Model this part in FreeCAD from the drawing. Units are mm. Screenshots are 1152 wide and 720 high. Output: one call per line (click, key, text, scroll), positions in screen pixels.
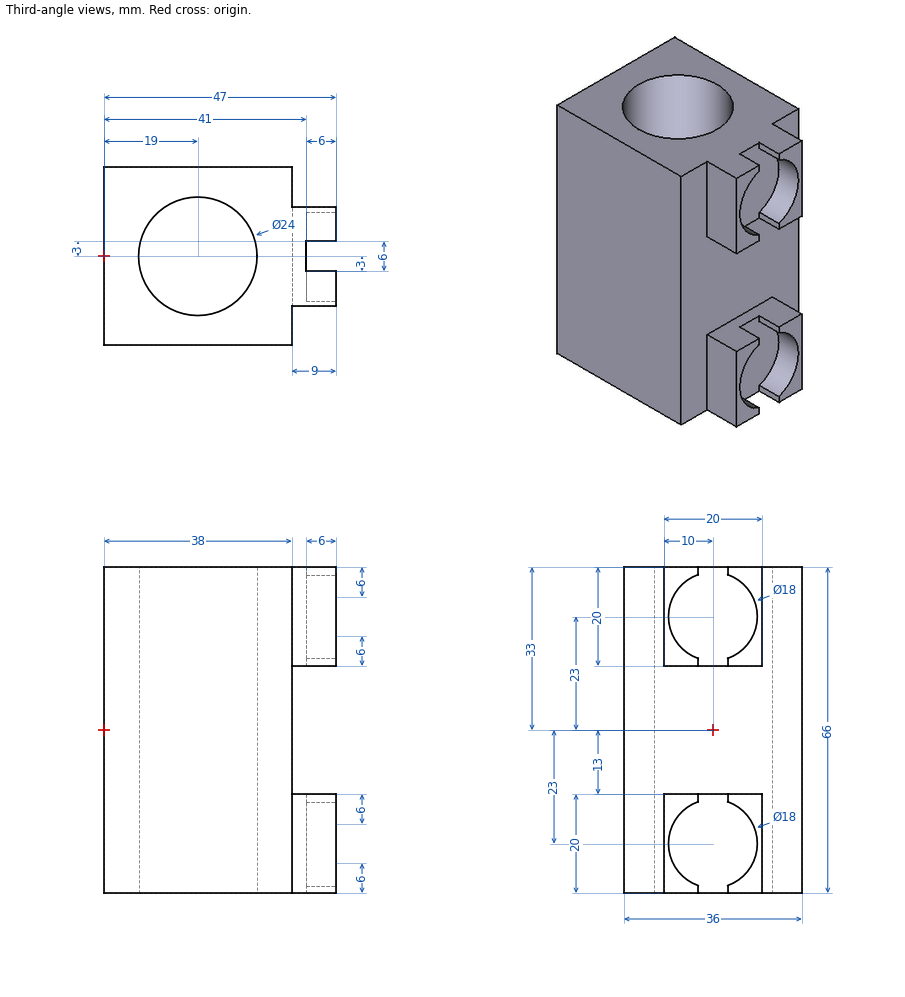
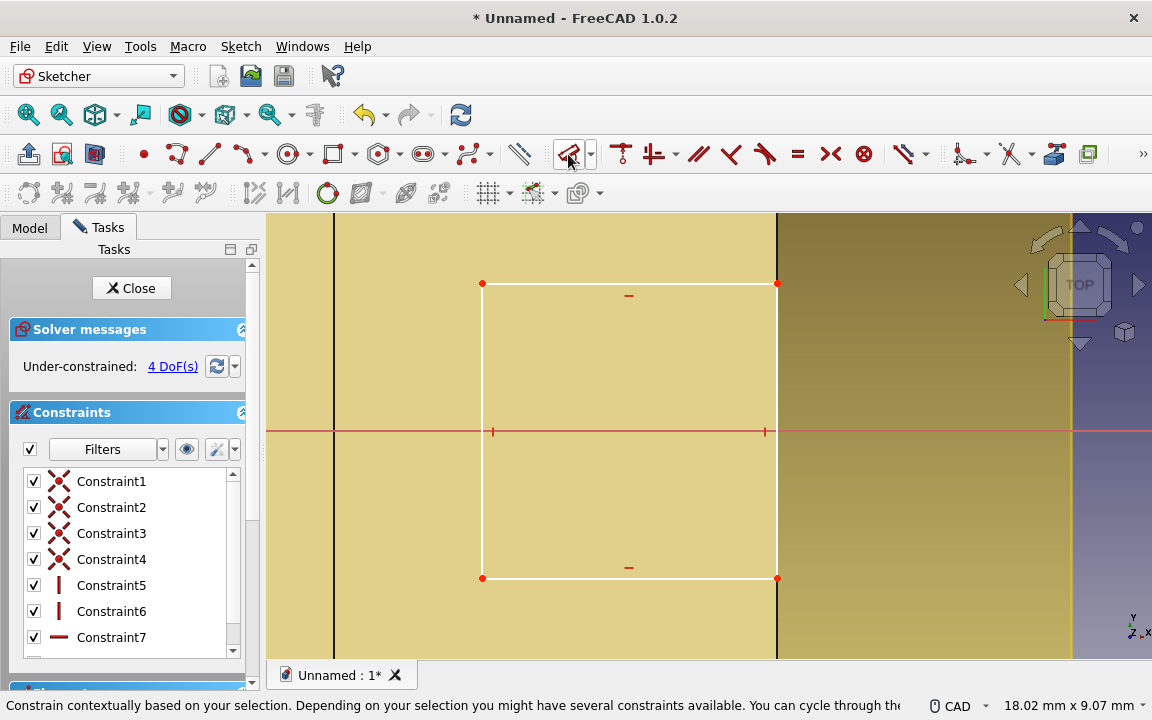
click(482, 373)
click(448, 364)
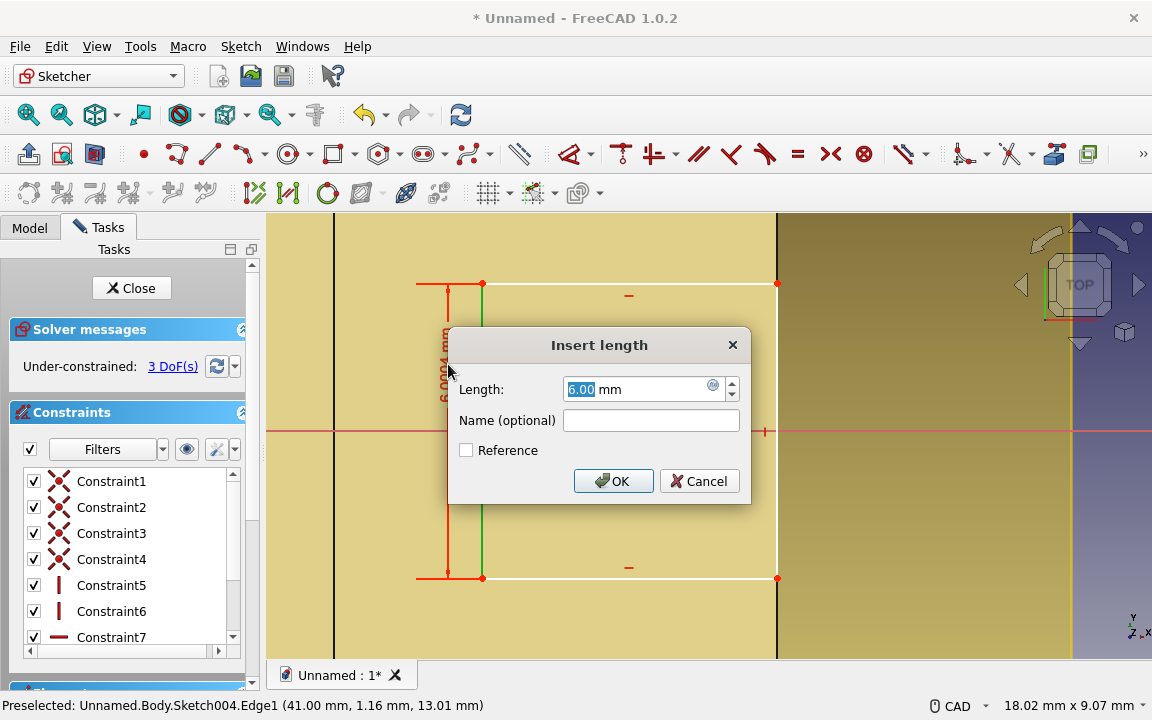
text(6)
key(Return)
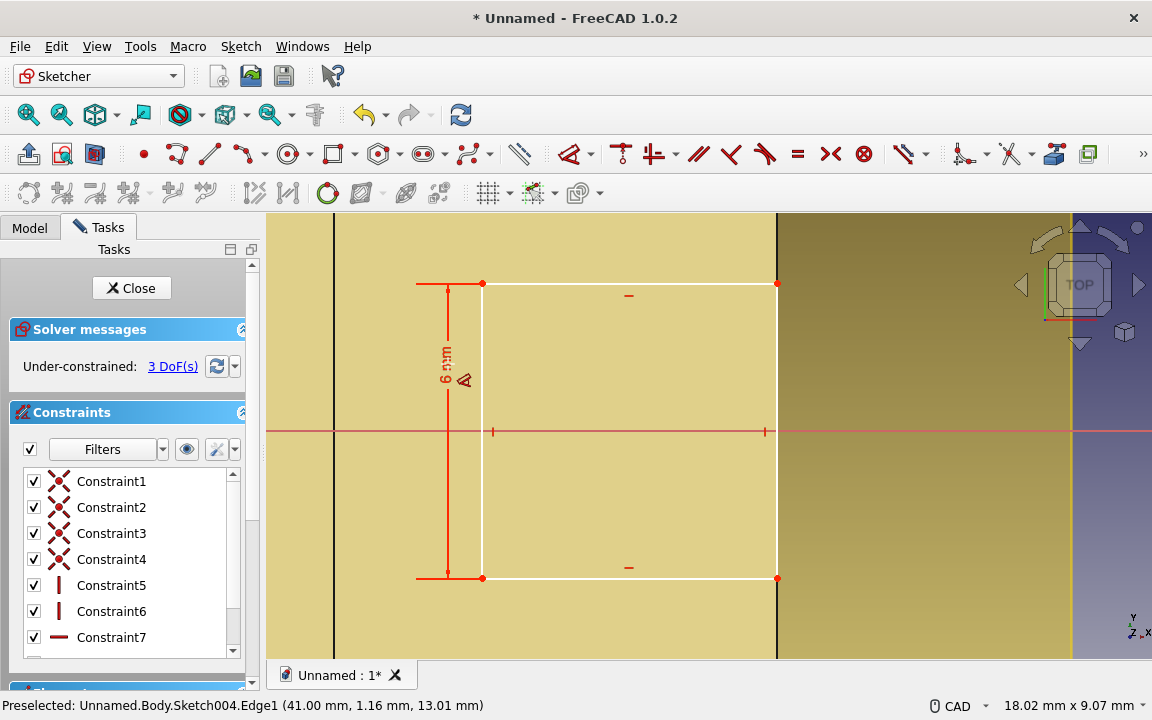
click(571, 579)
click(630, 613)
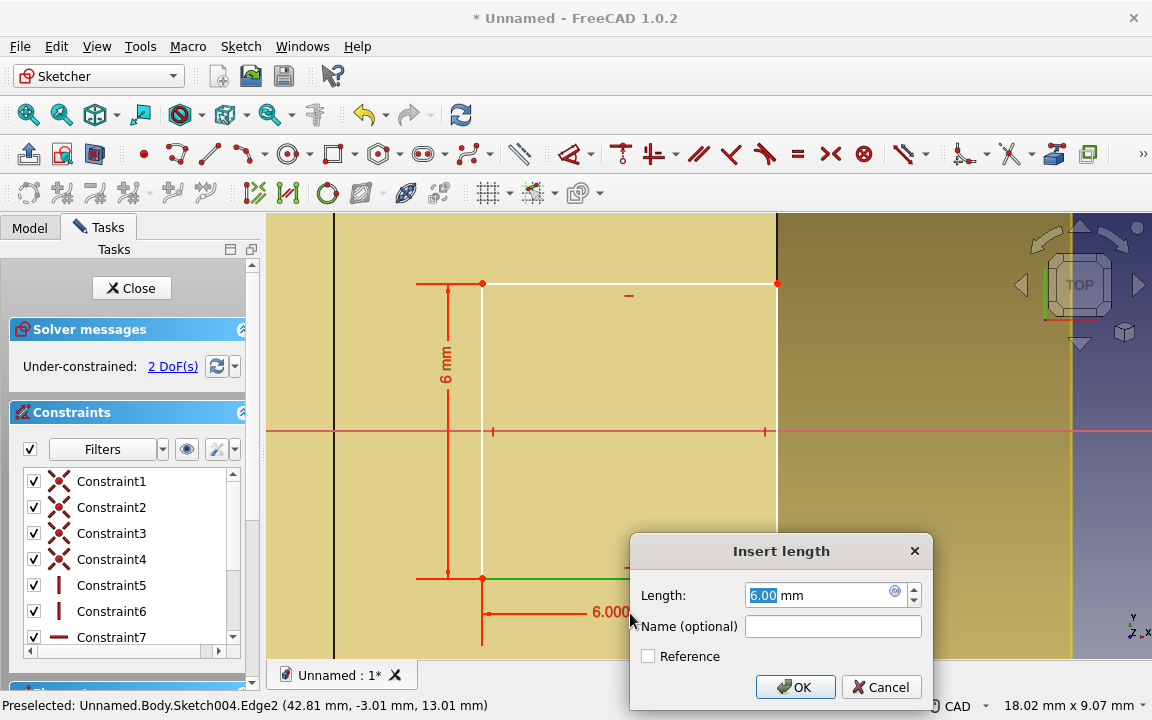
text(6)
key(Return)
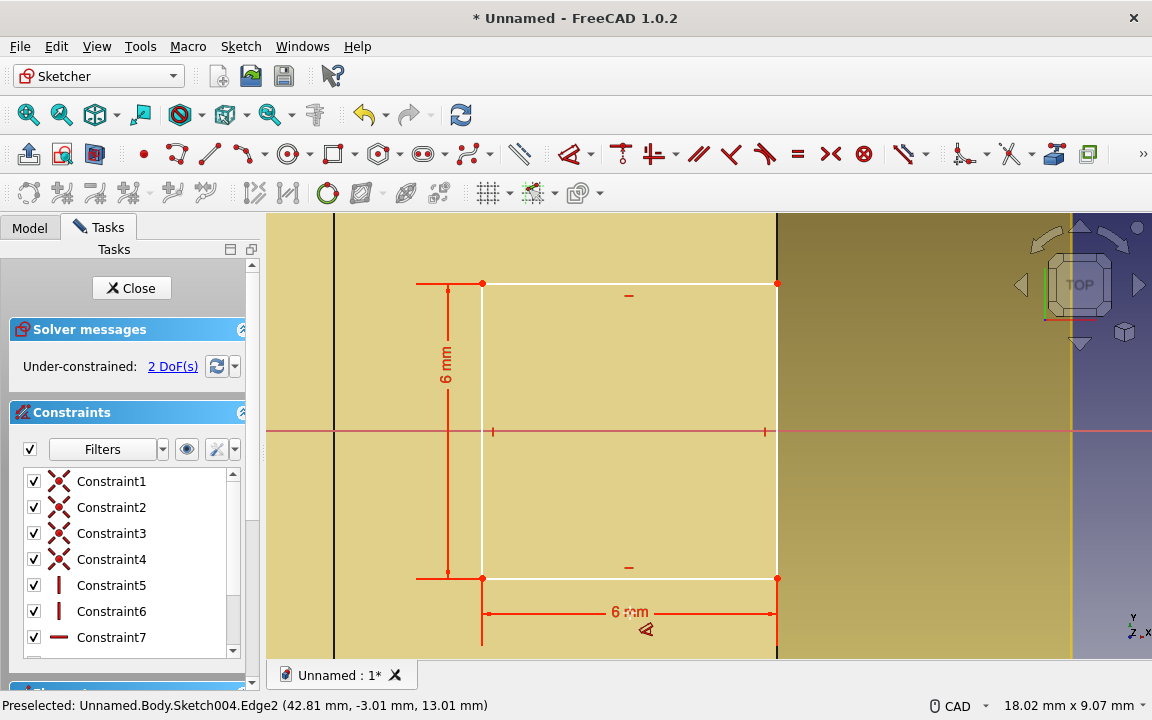
click(482, 284)
click(516, 324)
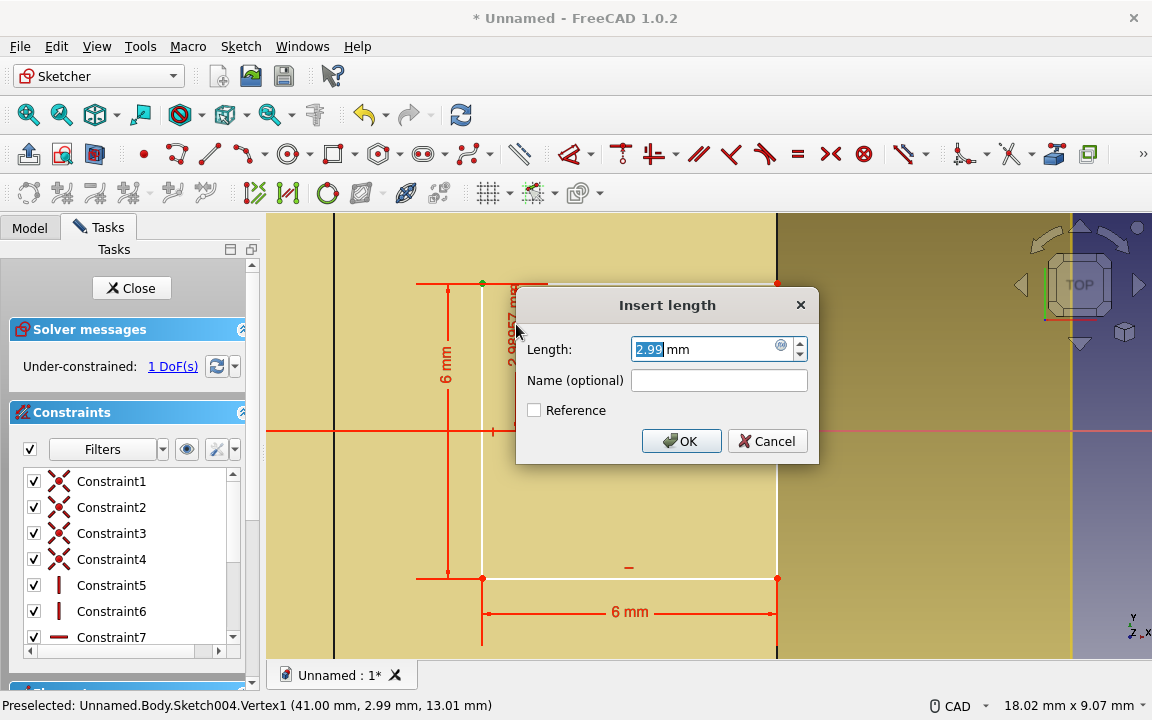
text(3)
key(Return)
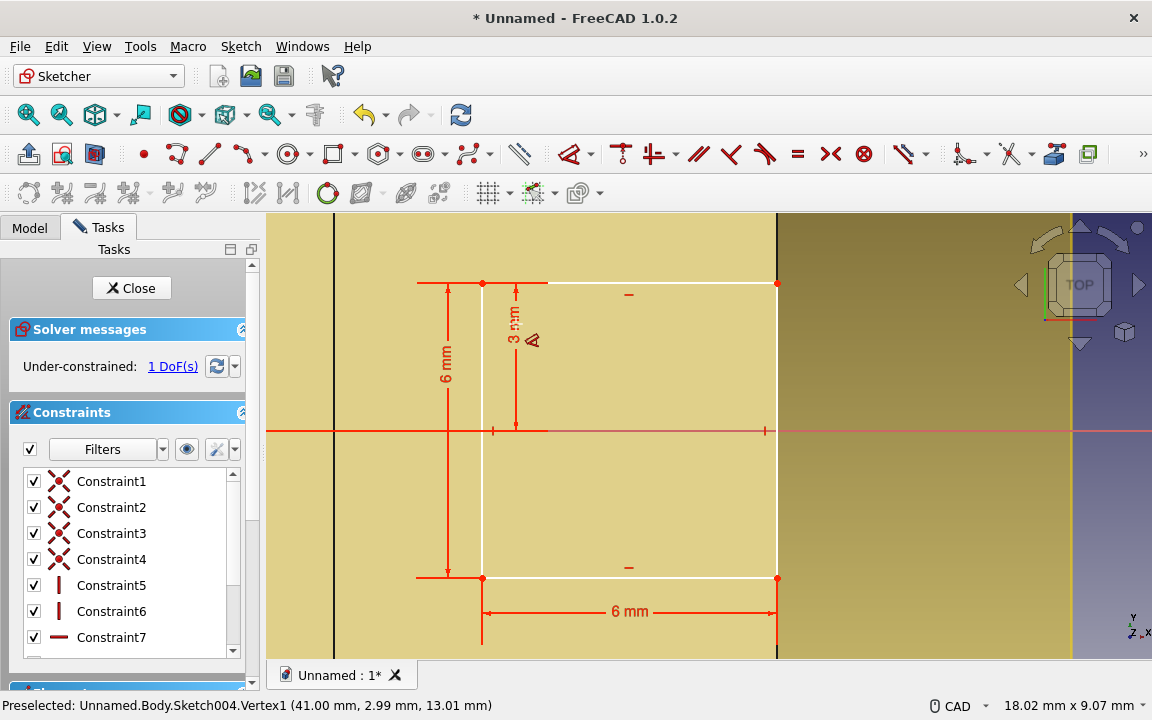
click(482, 283)
click(388, 249)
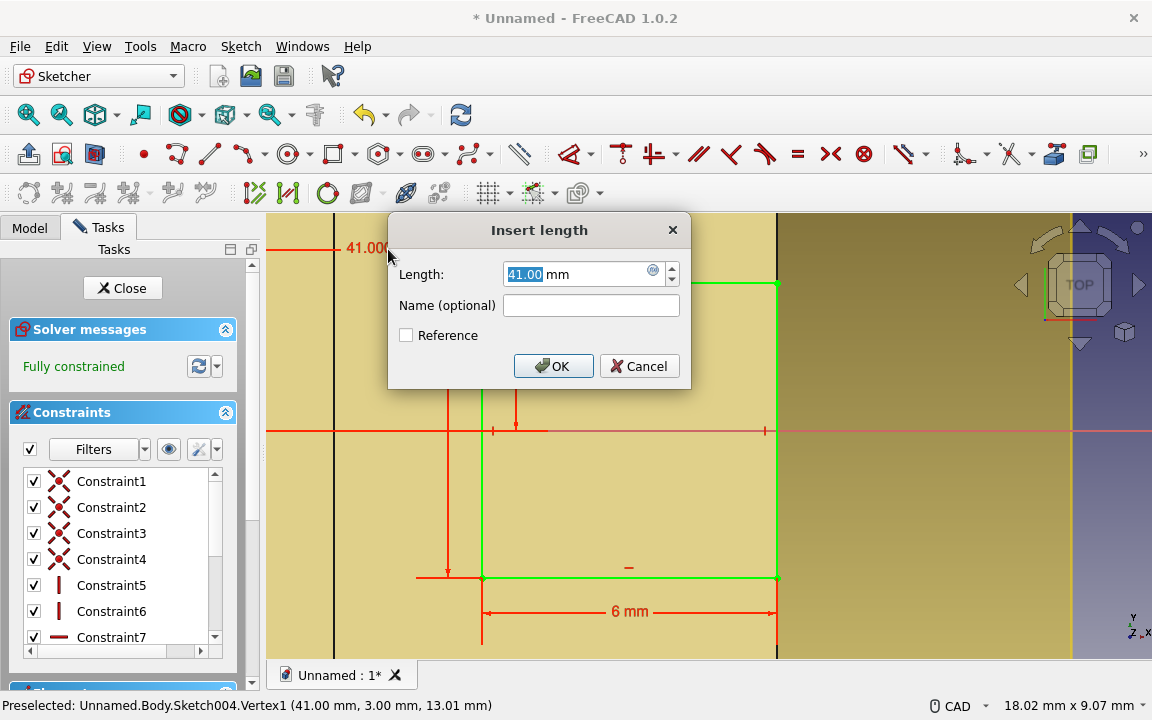
text(41)
key(Return)
key(Escape)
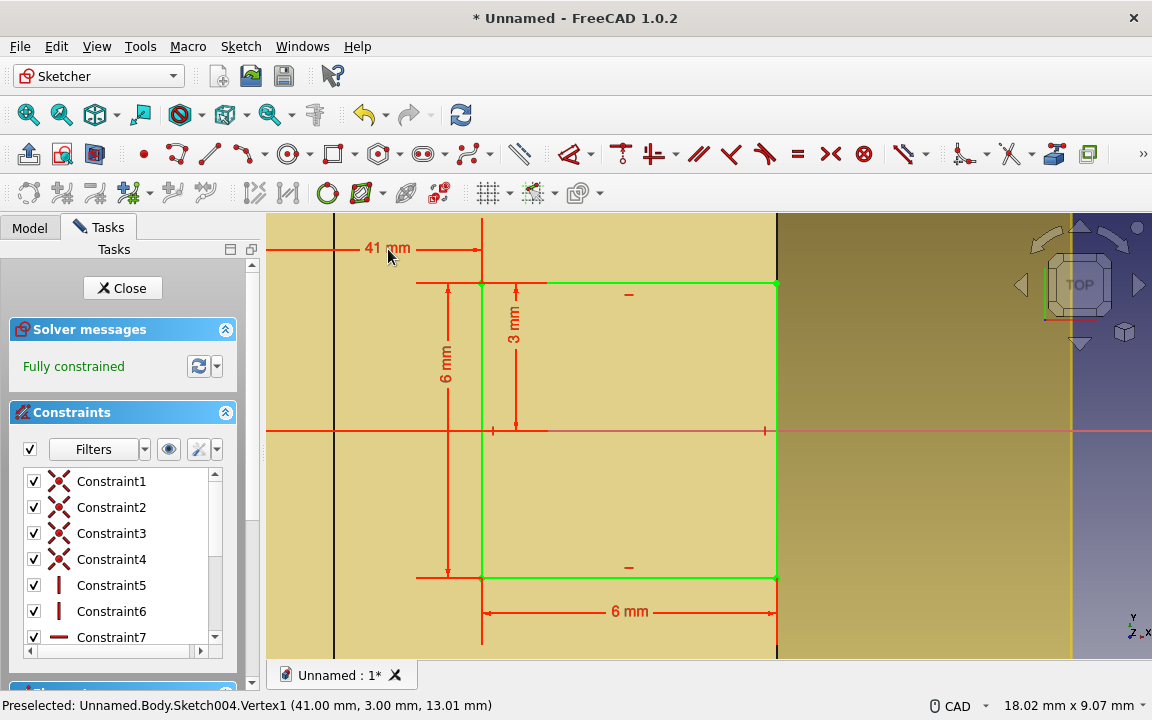
click(123, 288)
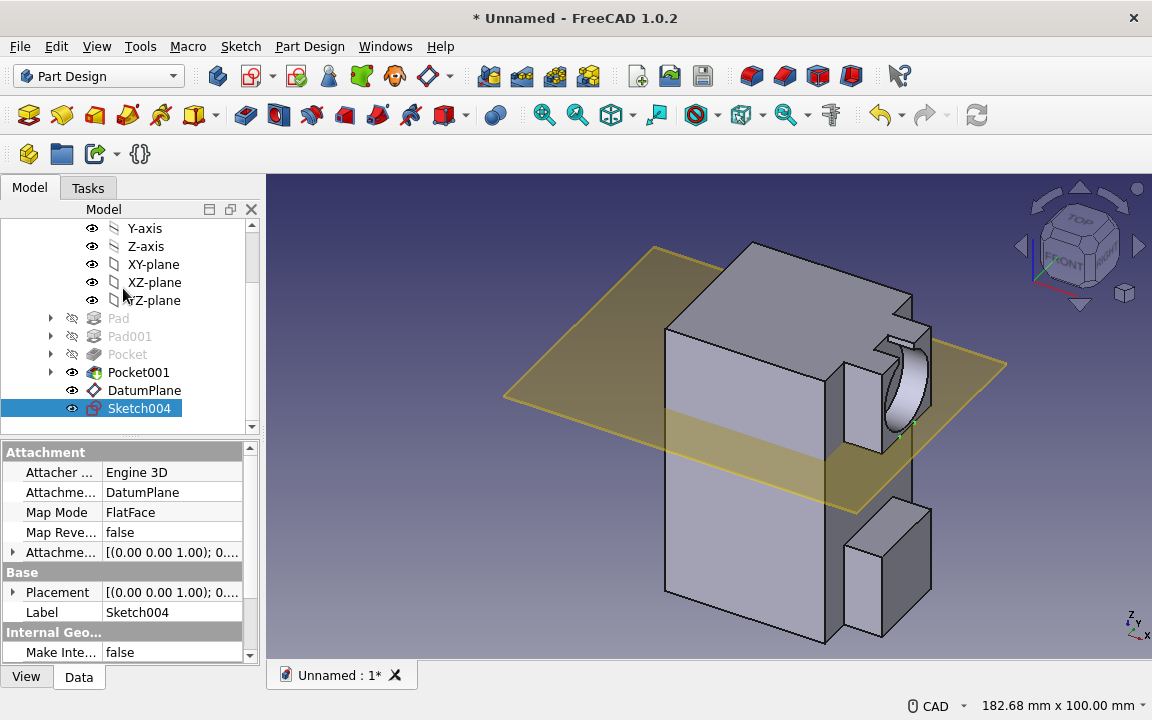
click(246, 116)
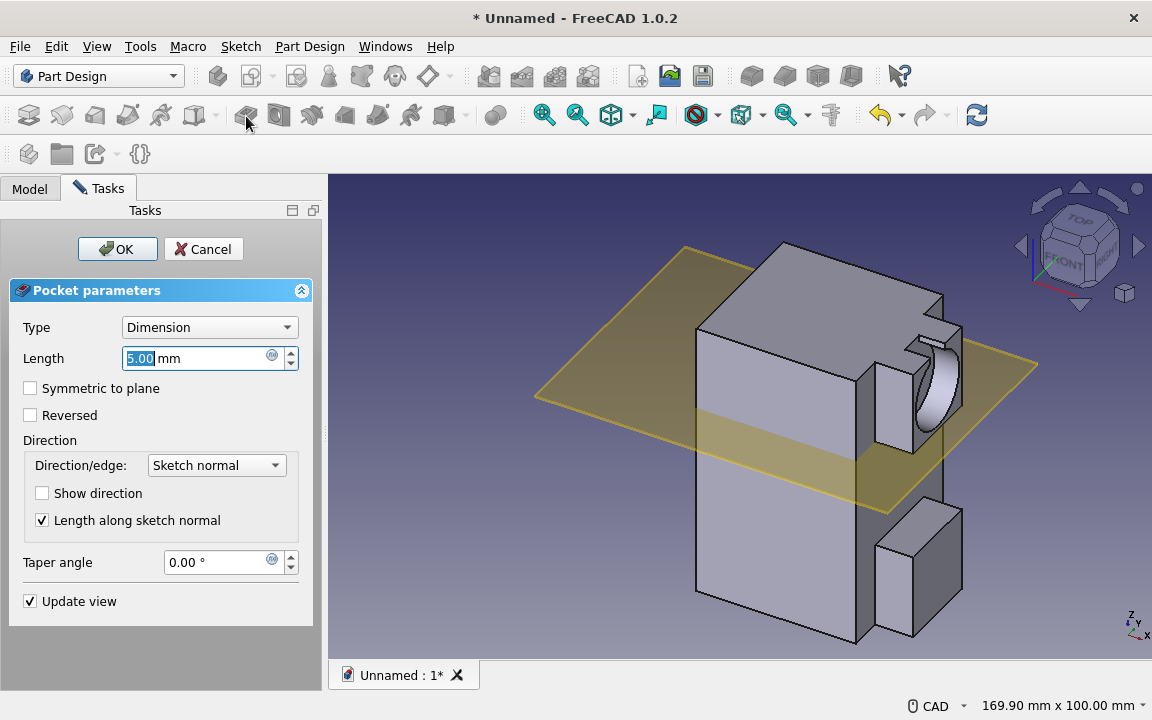
text(6)
key(Tab)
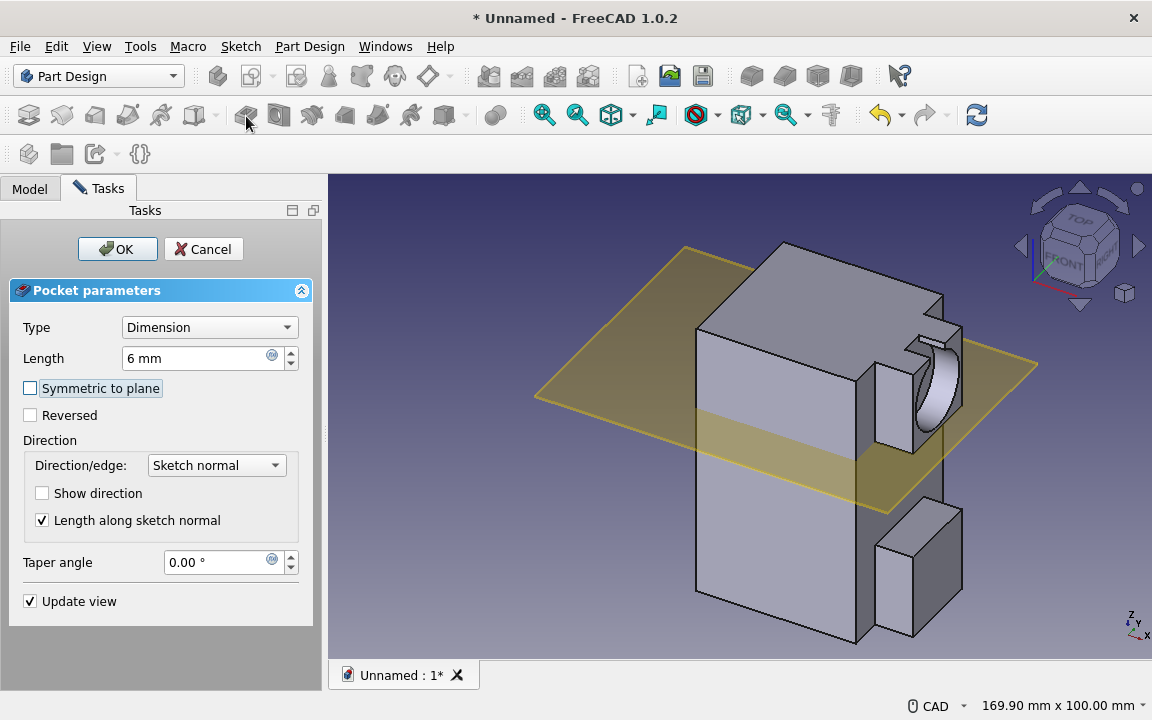
click(31, 415)